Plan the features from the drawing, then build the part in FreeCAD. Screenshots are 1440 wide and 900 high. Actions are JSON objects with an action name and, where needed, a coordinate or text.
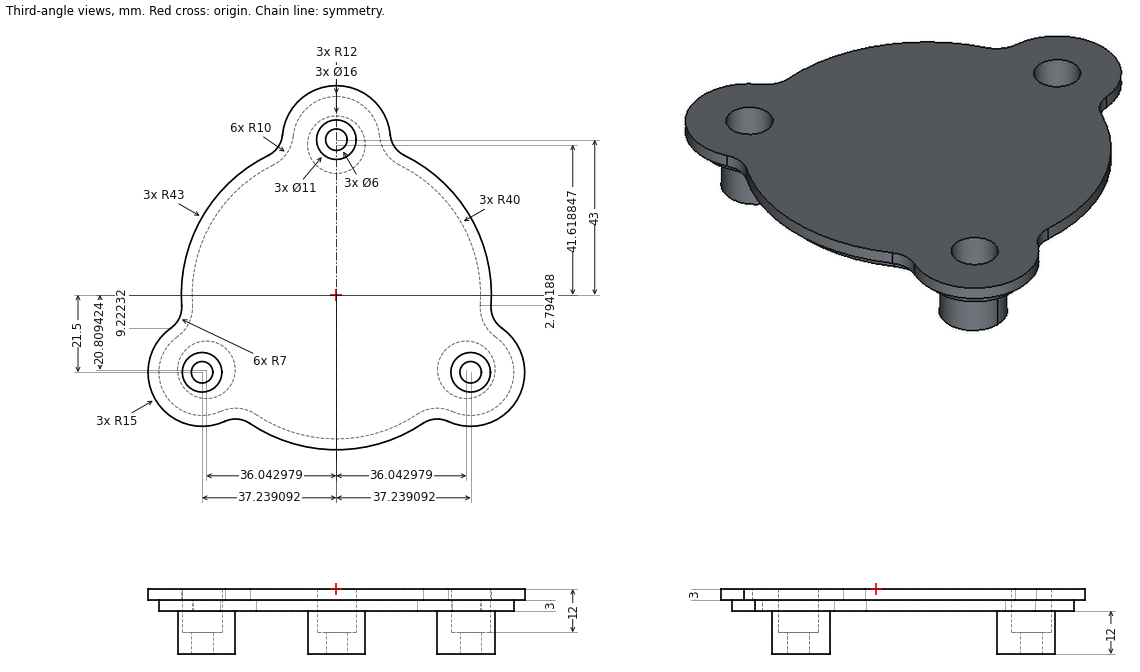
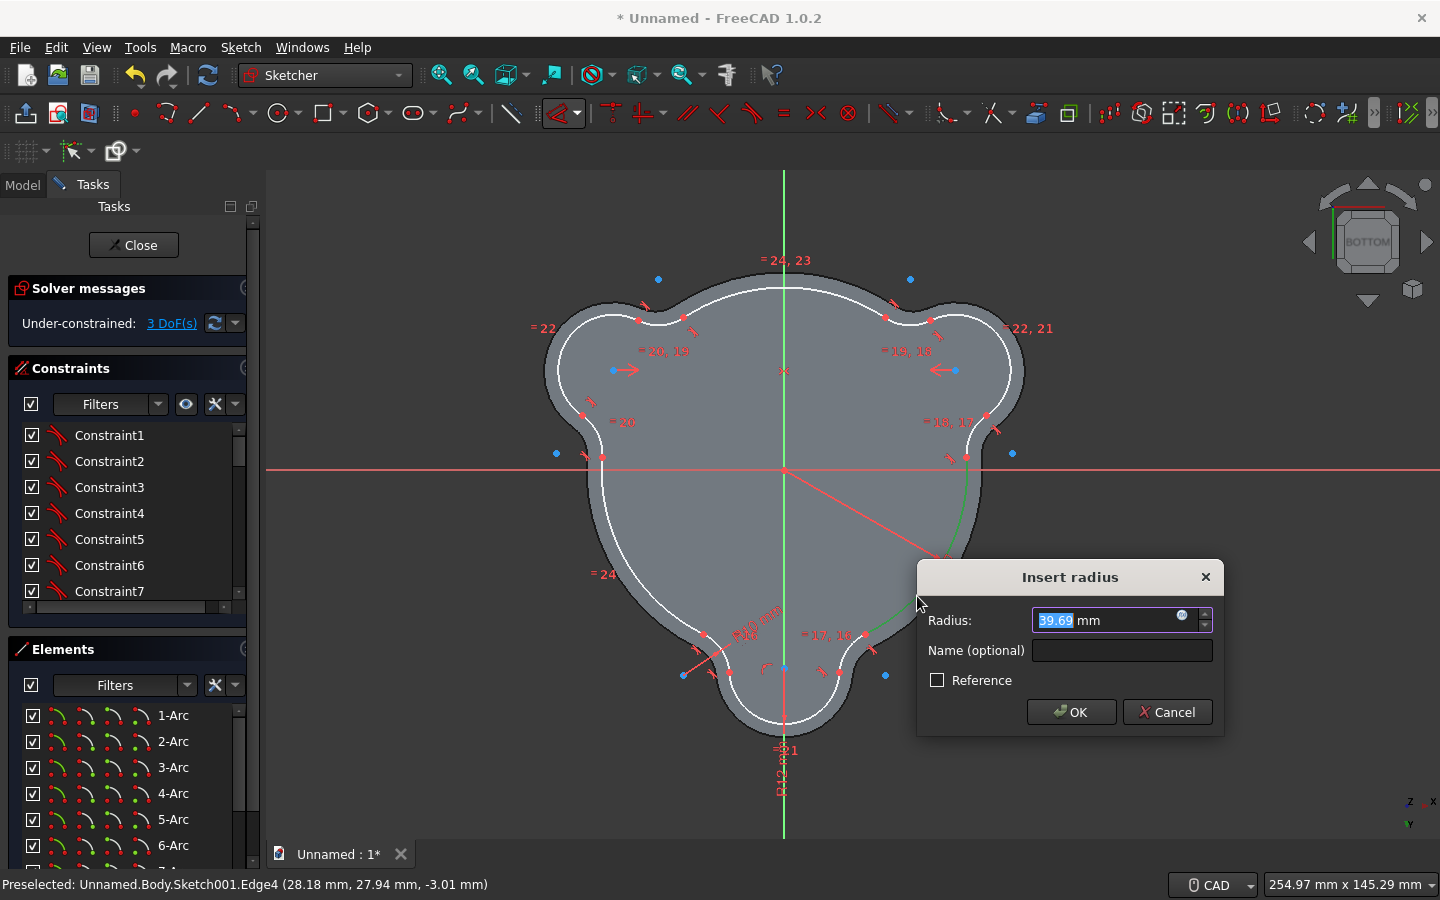
{"action": "type", "text": "40"}
{"action": "key", "text": "Return"}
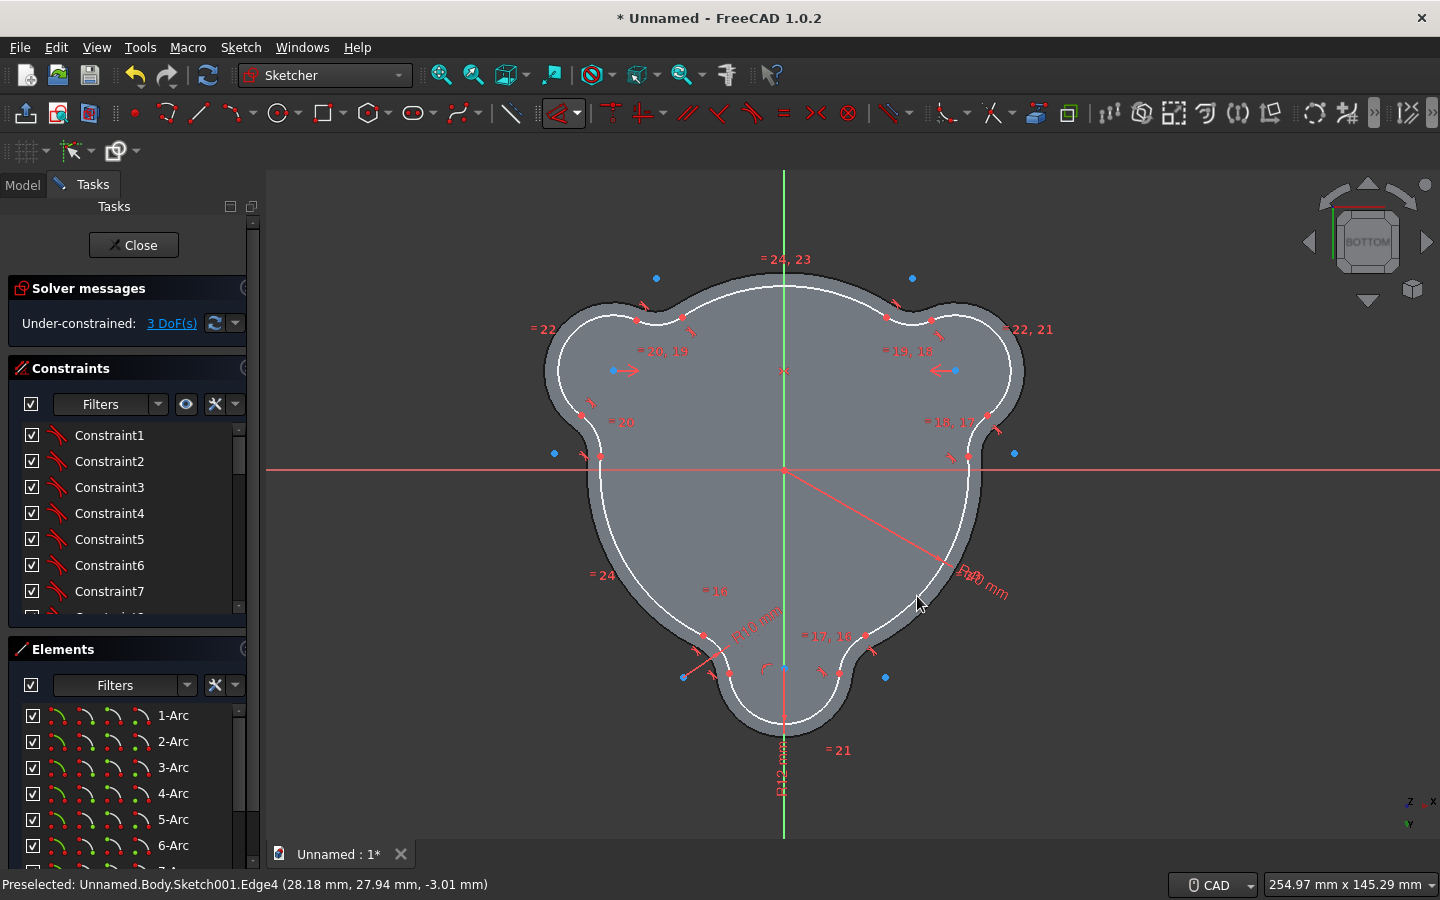
{"action": "left_click", "coordinate": [784, 669]}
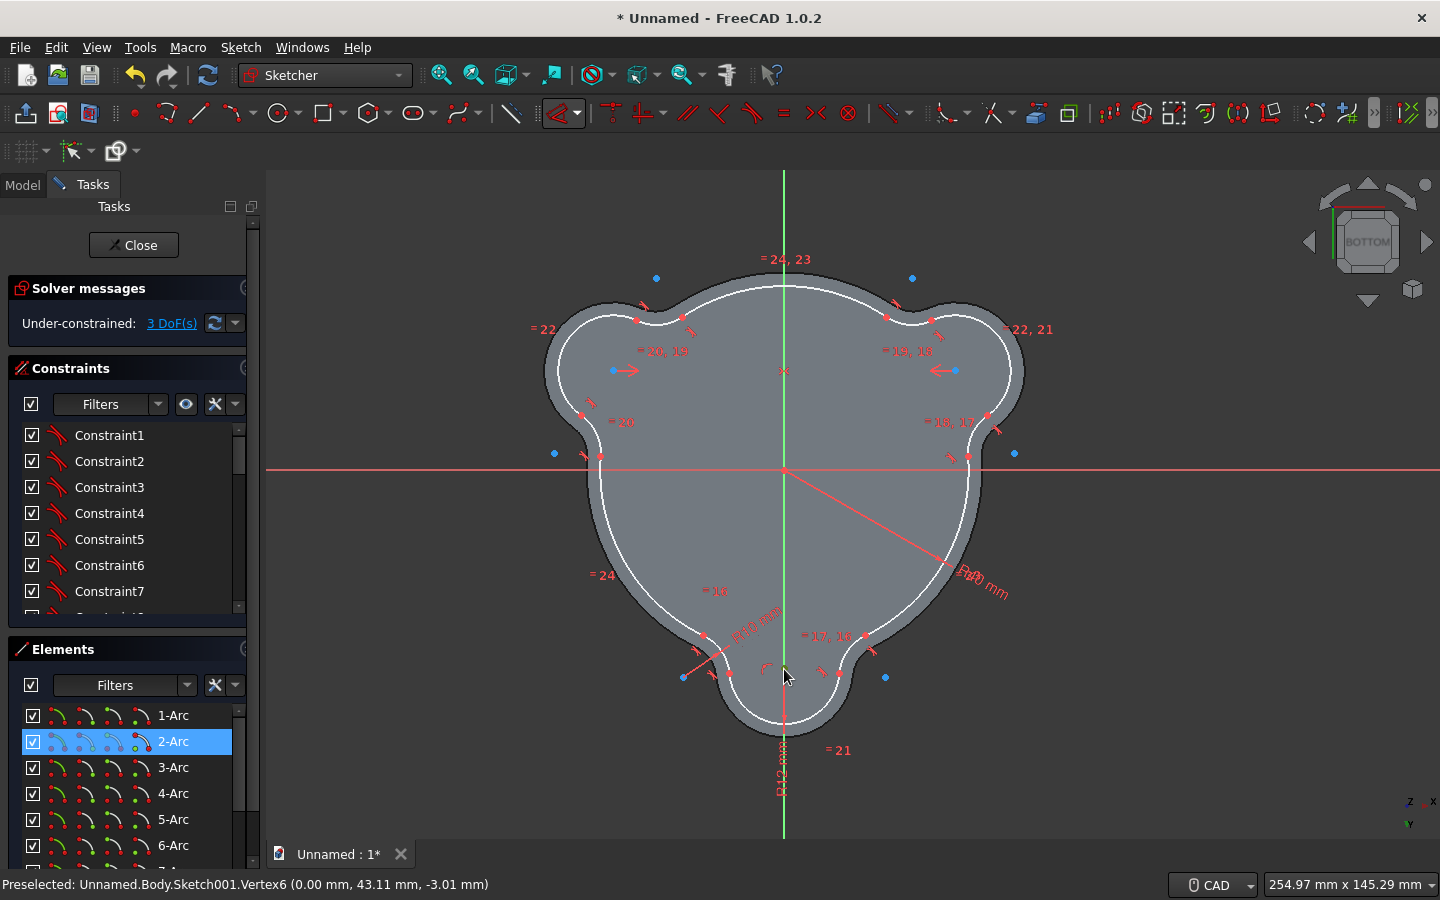
{"action": "left_click", "coordinate": [580, 114]}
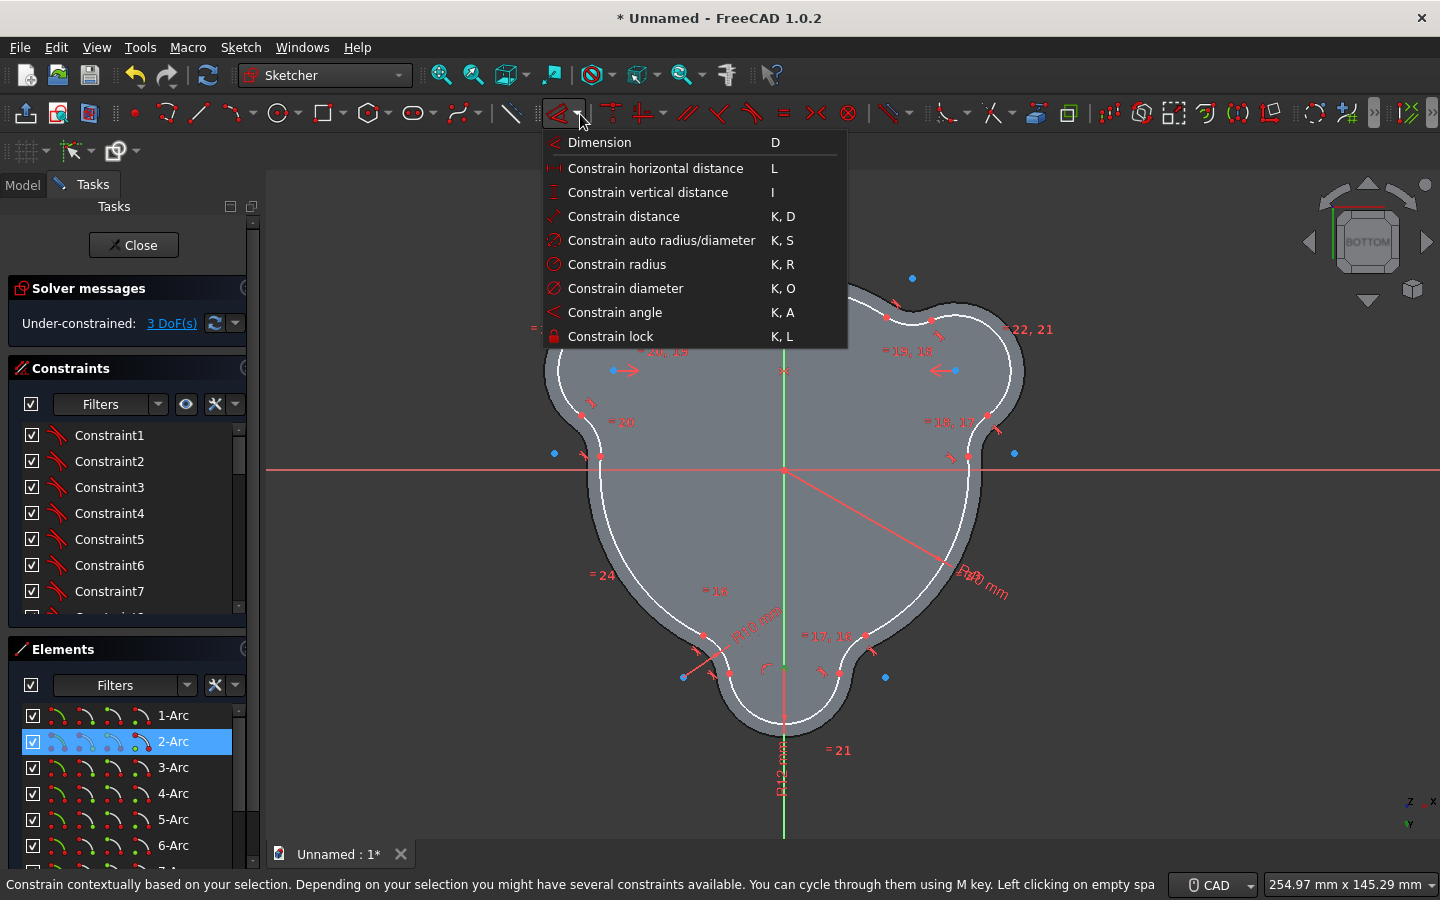
{"action": "left_click", "coordinate": [695, 192]}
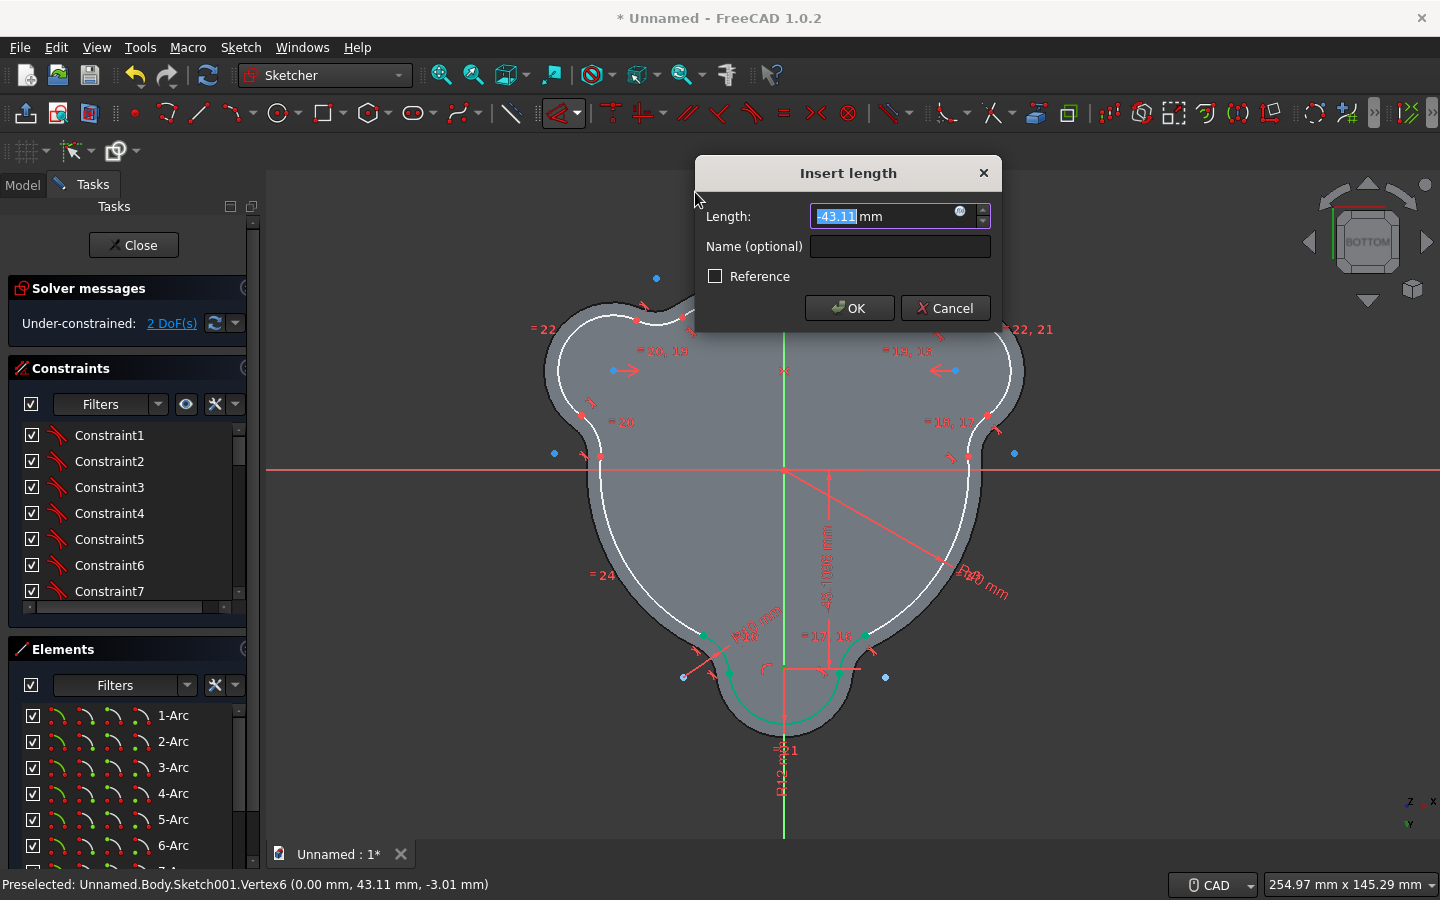
{"action": "type", "text": "-43"}
{"action": "key", "text": "Return"}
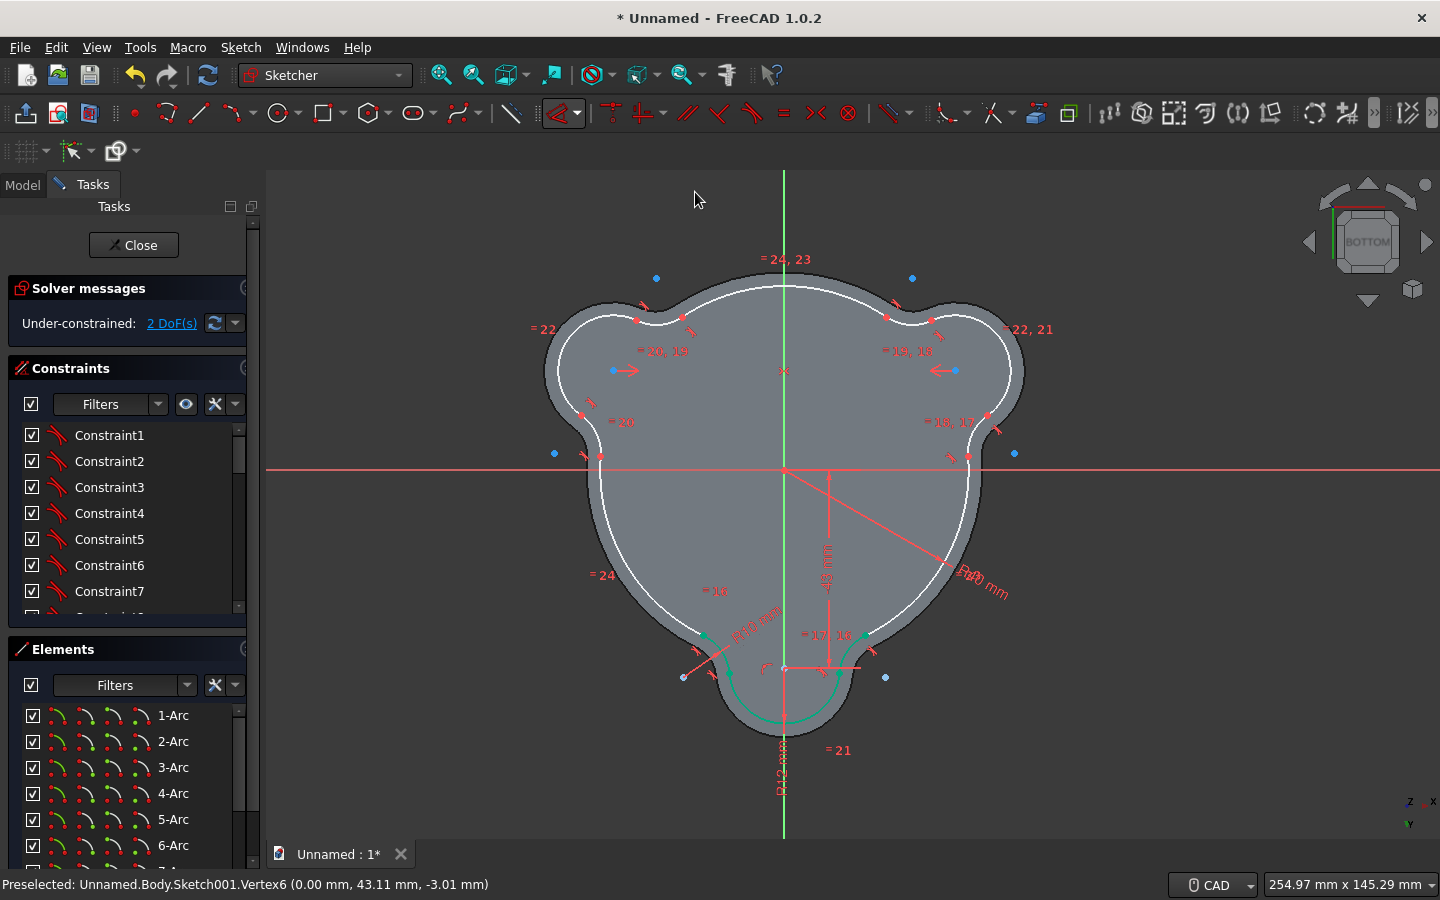
{"action": "left_click", "coordinate": [955, 371]}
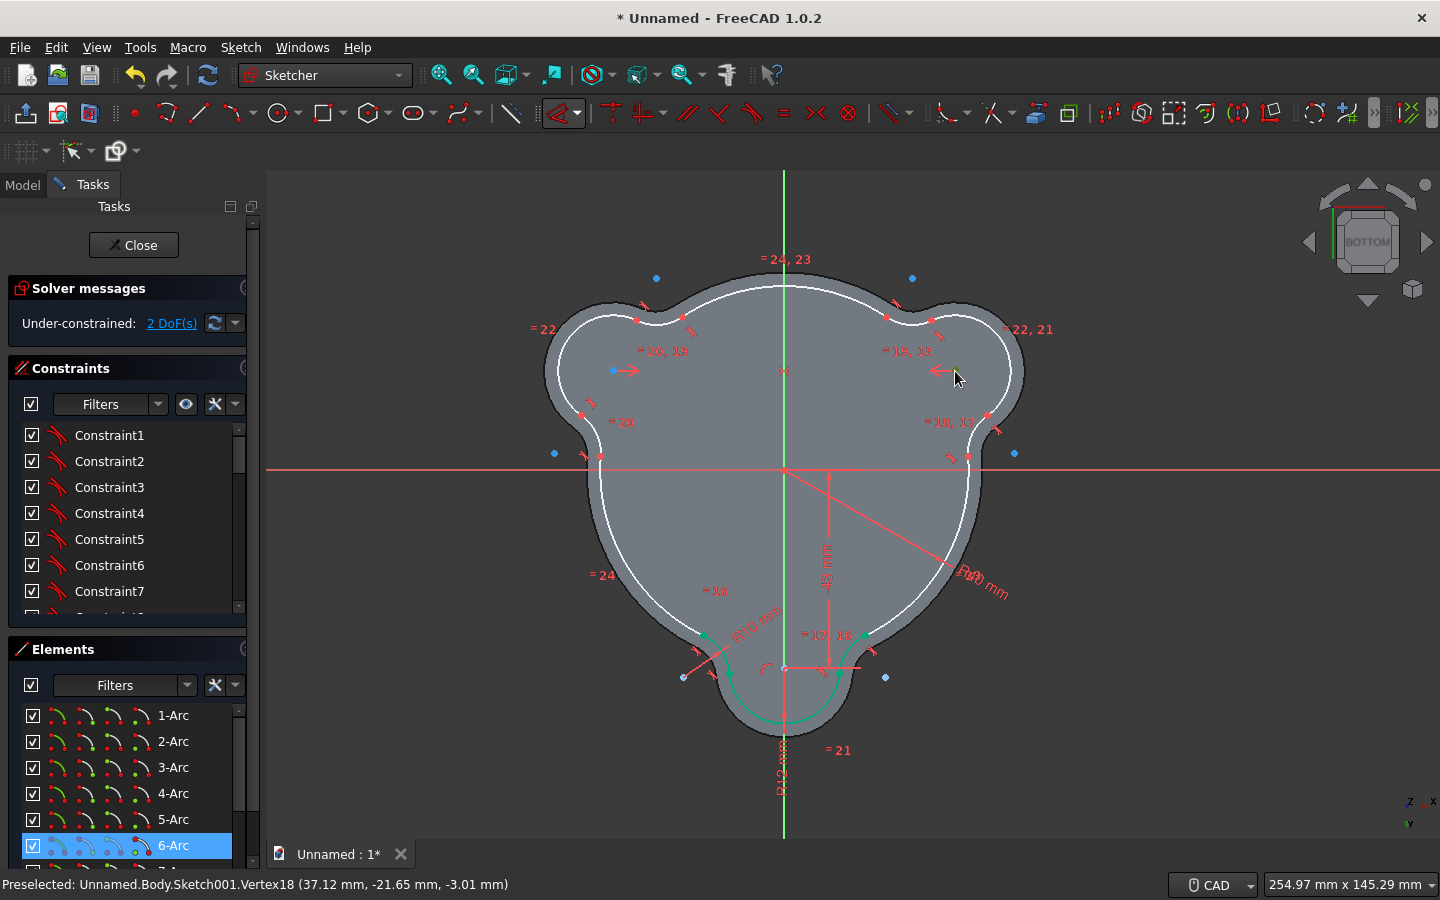
{"action": "key", "text": "i"}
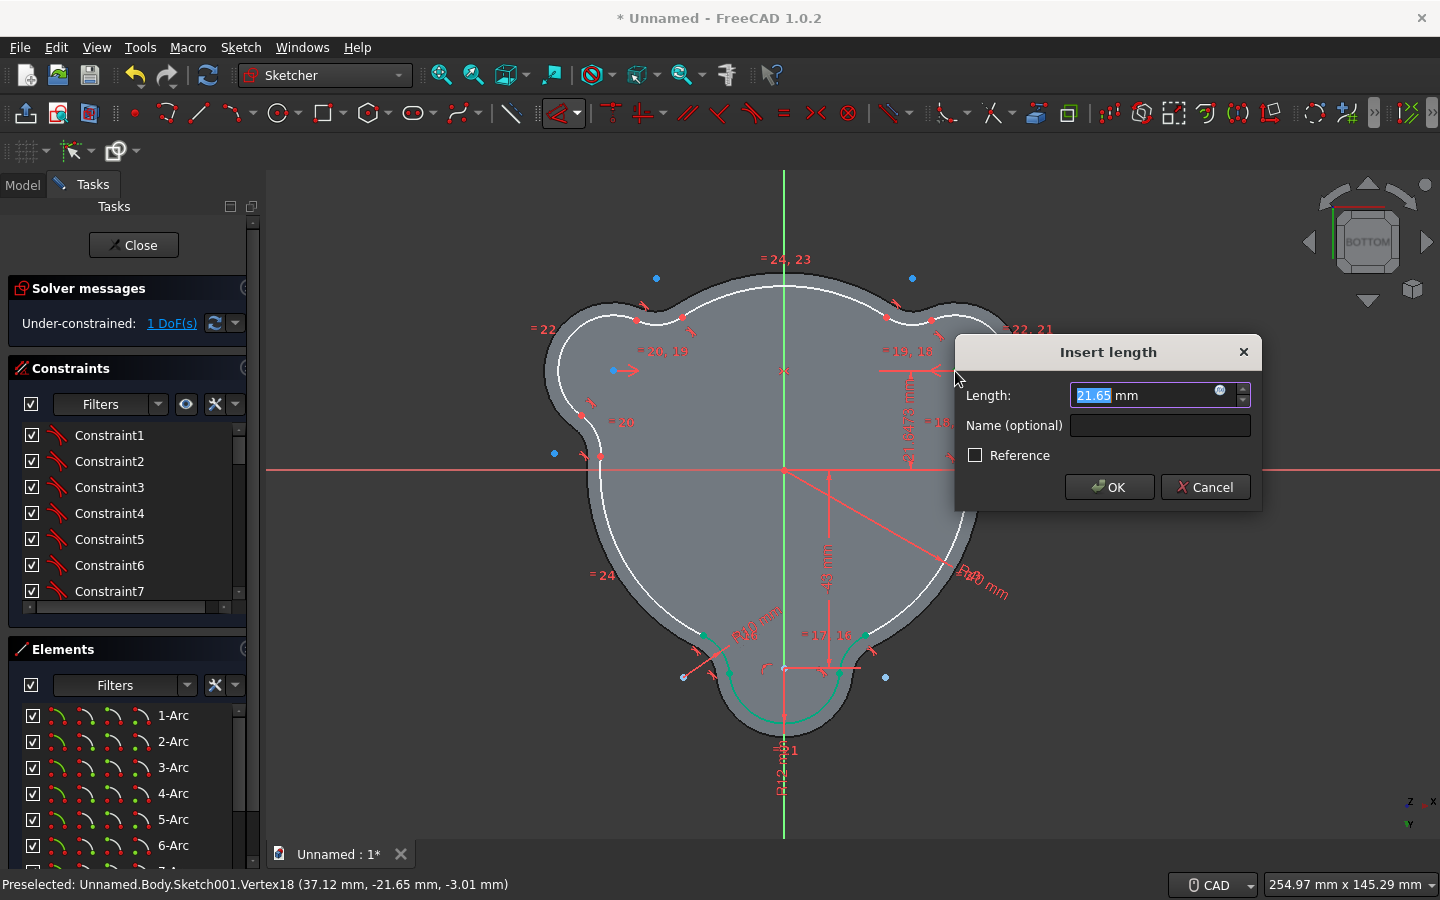
{"action": "type", "text": "21.5"}
{"action": "key", "text": "Return"}